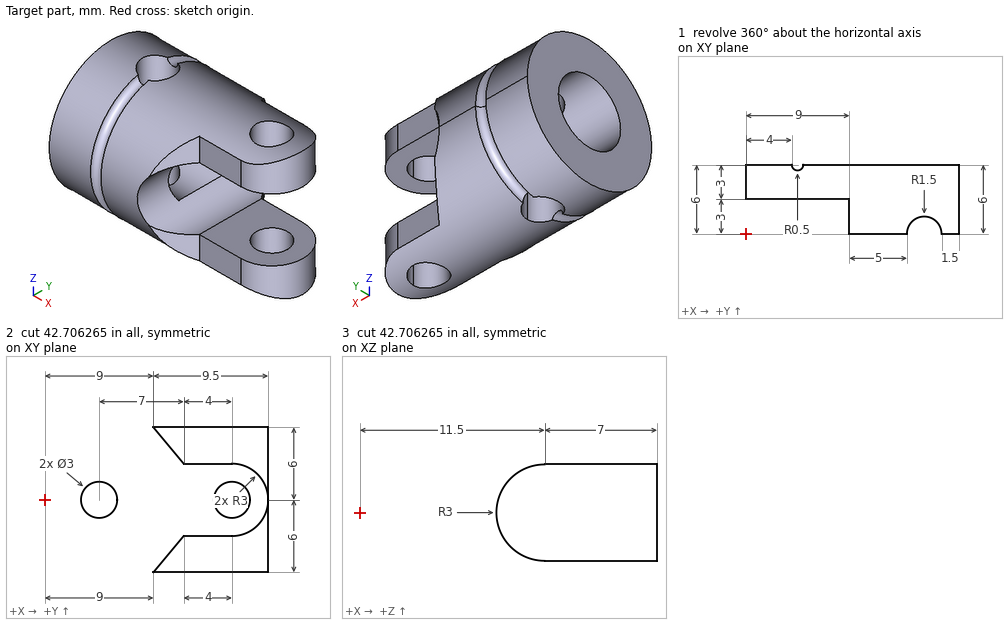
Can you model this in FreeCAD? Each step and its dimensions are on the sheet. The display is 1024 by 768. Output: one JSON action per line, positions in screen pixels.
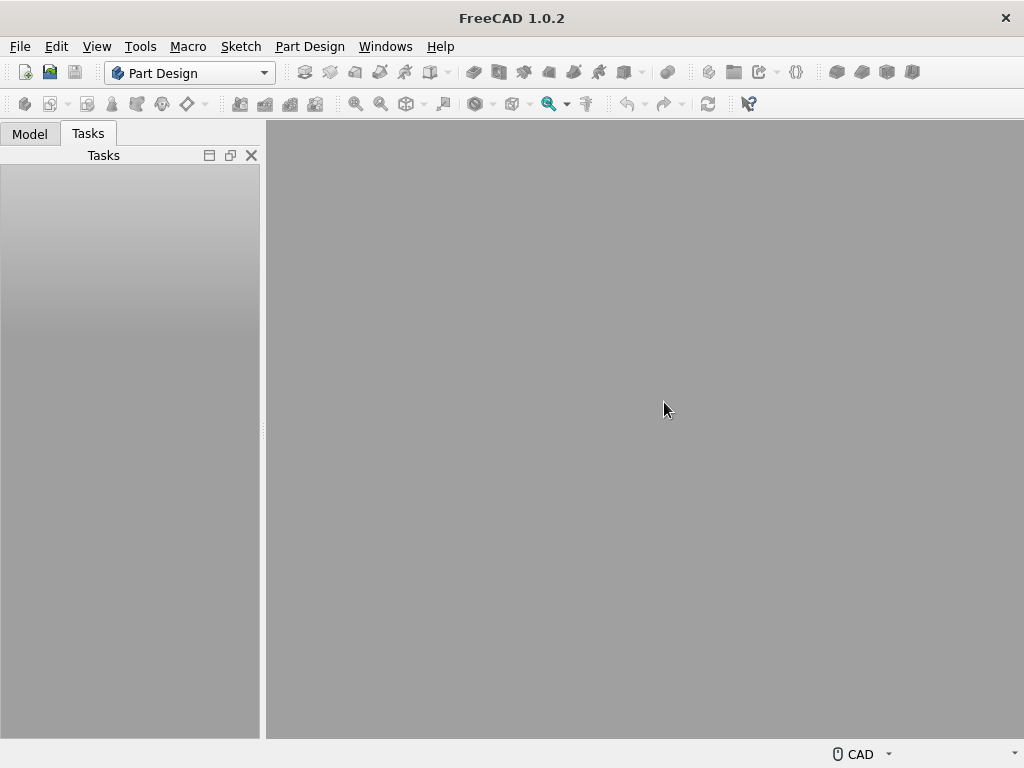
{"action": "left_click", "coordinate": [25, 72]}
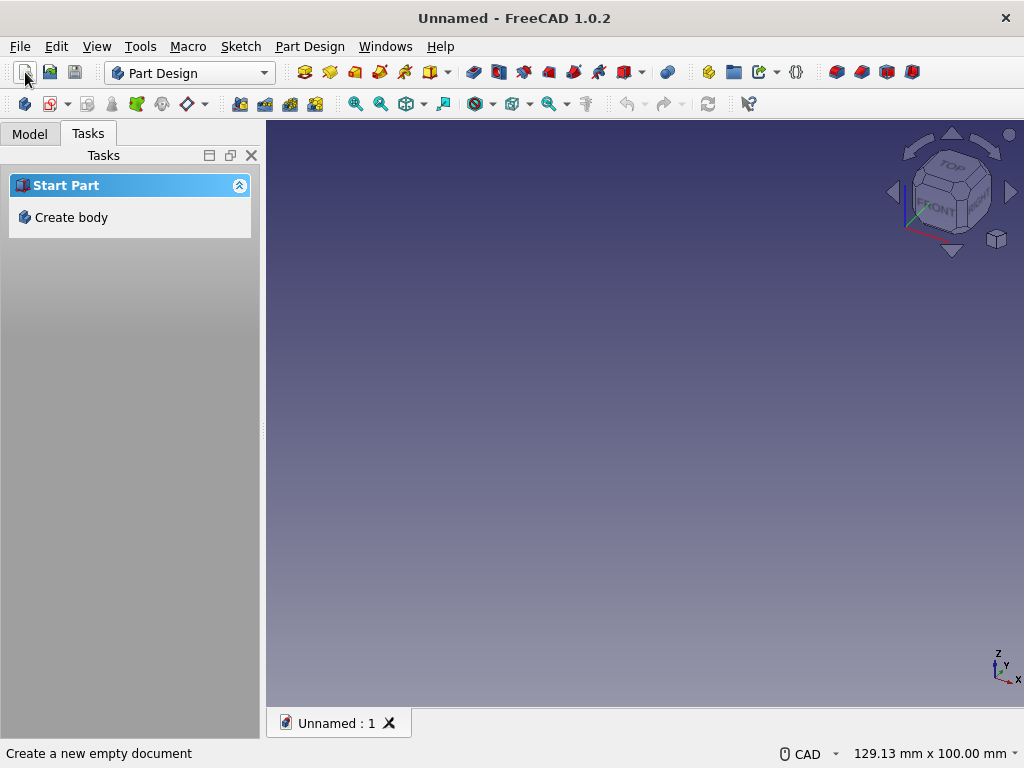
{"action": "left_click", "coordinate": [50, 104]}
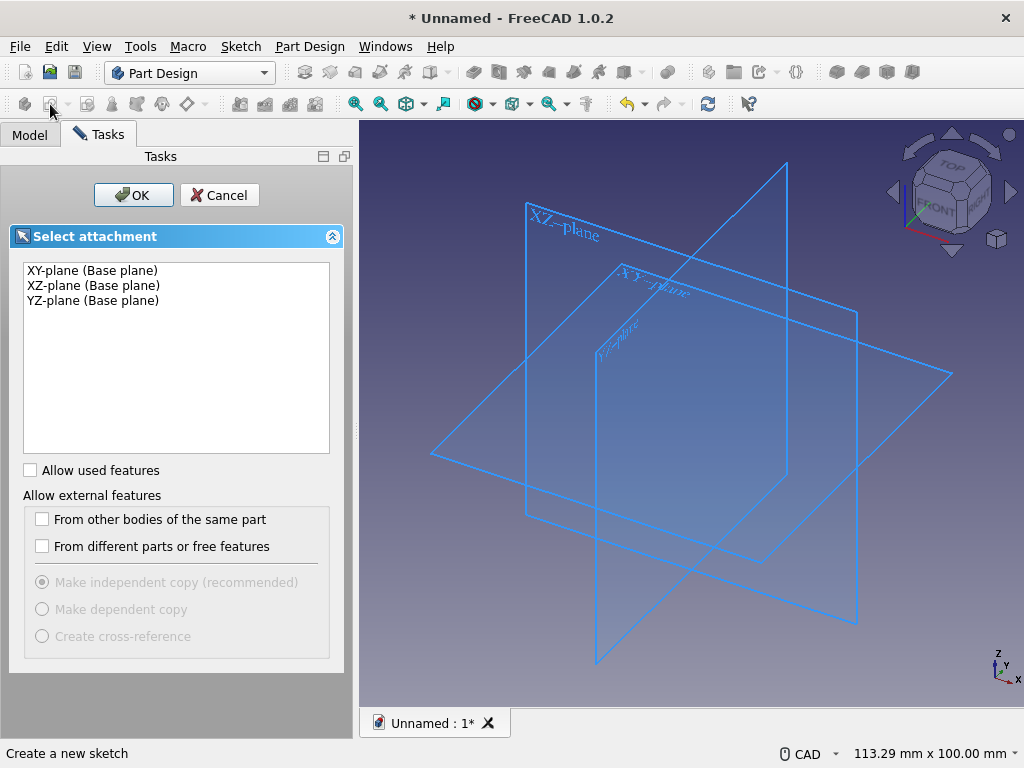
{"action": "left_click", "coordinate": [84, 270]}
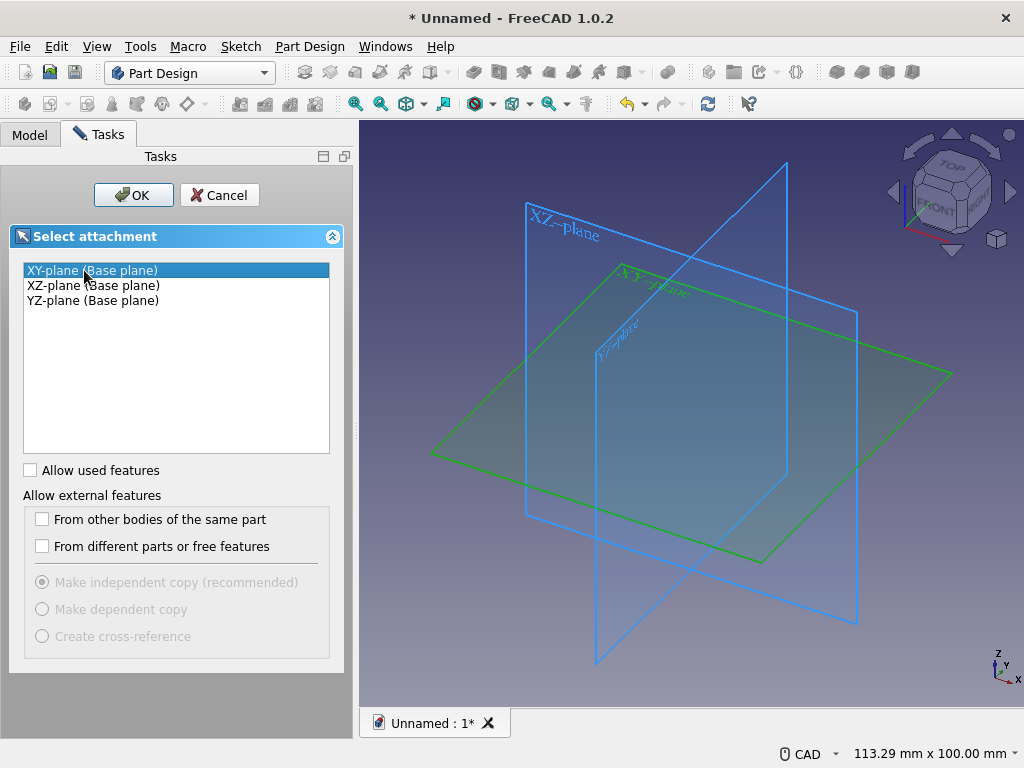
{"action": "left_click", "coordinate": [134, 195]}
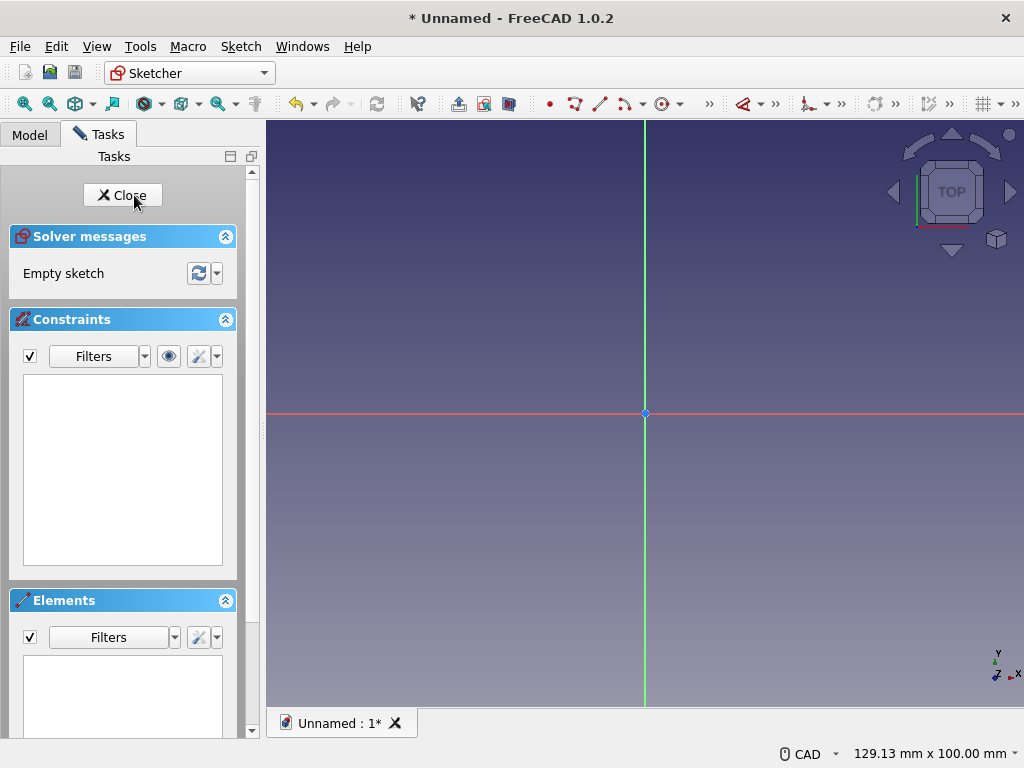
{"action": "scroll", "coordinate": [739, 390], "scroll_direction": "up", "scroll_amount": 7}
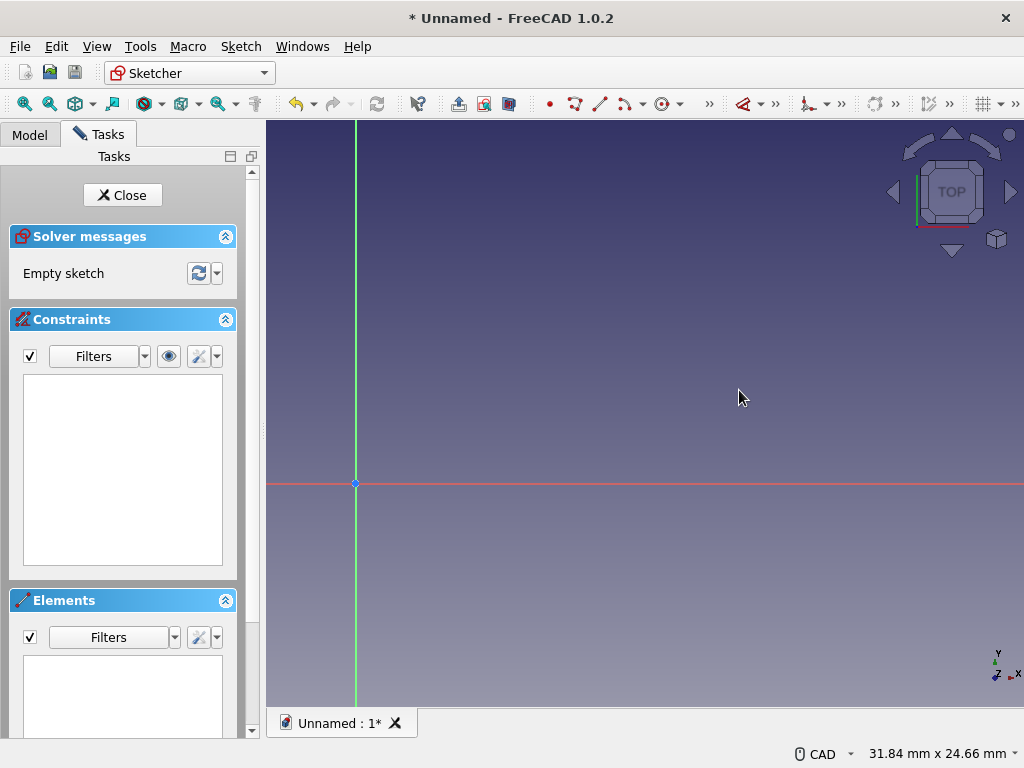
{"action": "left_click", "coordinate": [575, 104]}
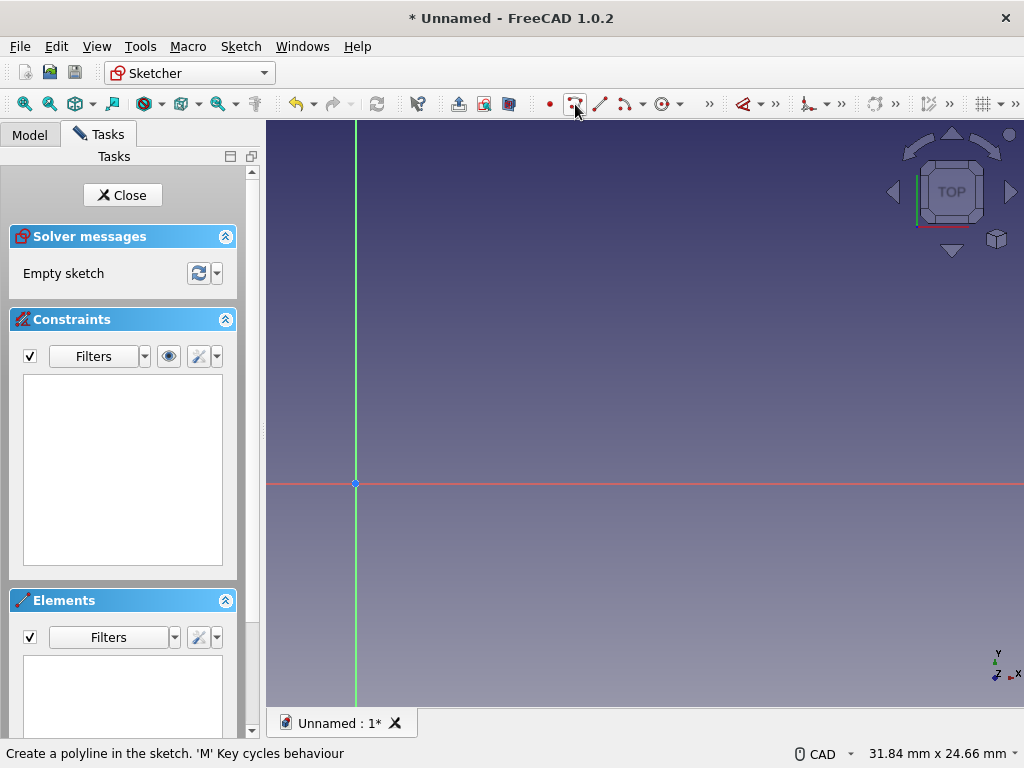
{"action": "left_click", "coordinate": [451, 341]}
{"action": "left_click", "coordinate": [356, 341]}
{"action": "left_click", "coordinate": [365, 412]}
{"action": "left_click", "coordinate": [570, 412]}
{"action": "left_click", "coordinate": [570, 484]}
{"action": "left_click", "coordinate": [689, 475]}
{"action": "right_click", "coordinate": [689, 475]}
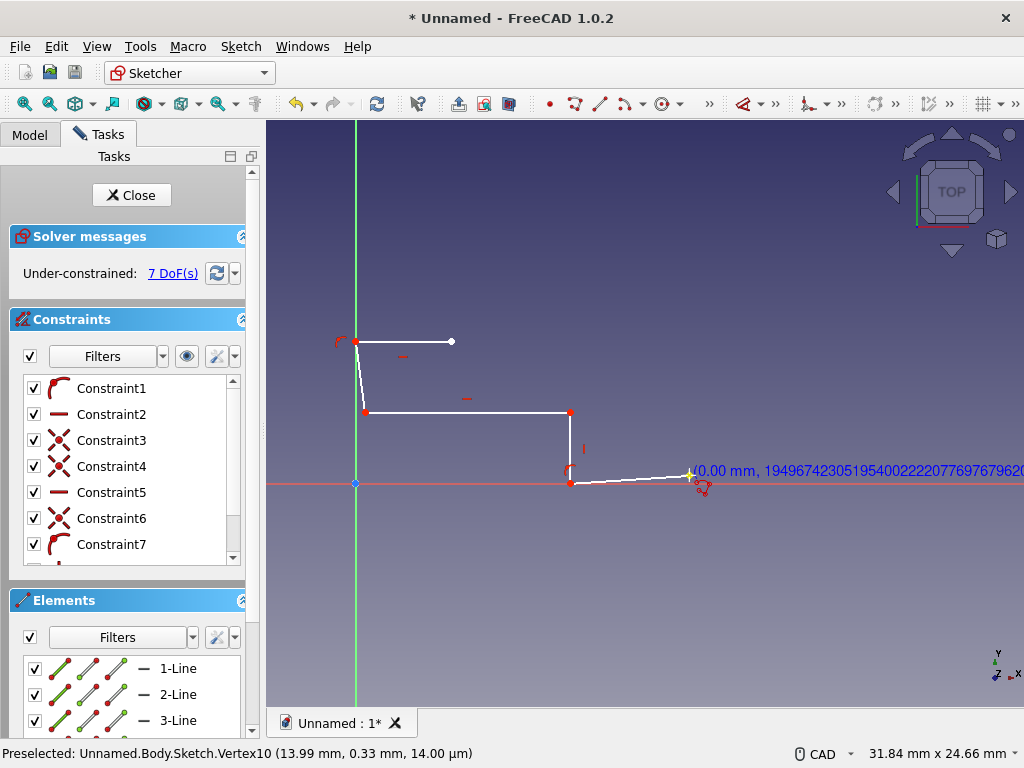
{"action": "left_click", "coordinate": [761, 484]}
{"action": "left_click", "coordinate": [796, 475]}
{"action": "left_click", "coordinate": [796, 341]}
{"action": "left_click", "coordinate": [475, 341]}
{"action": "right_click", "coordinate": [475, 341]}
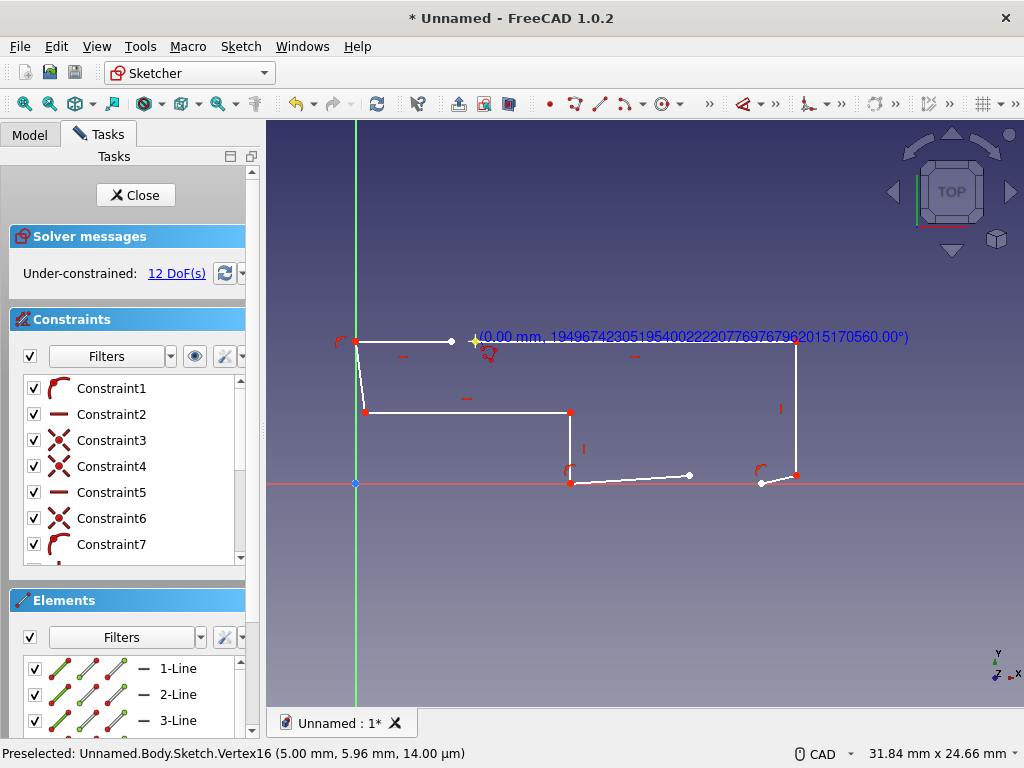
{"action": "key", "text": "g 3 a"}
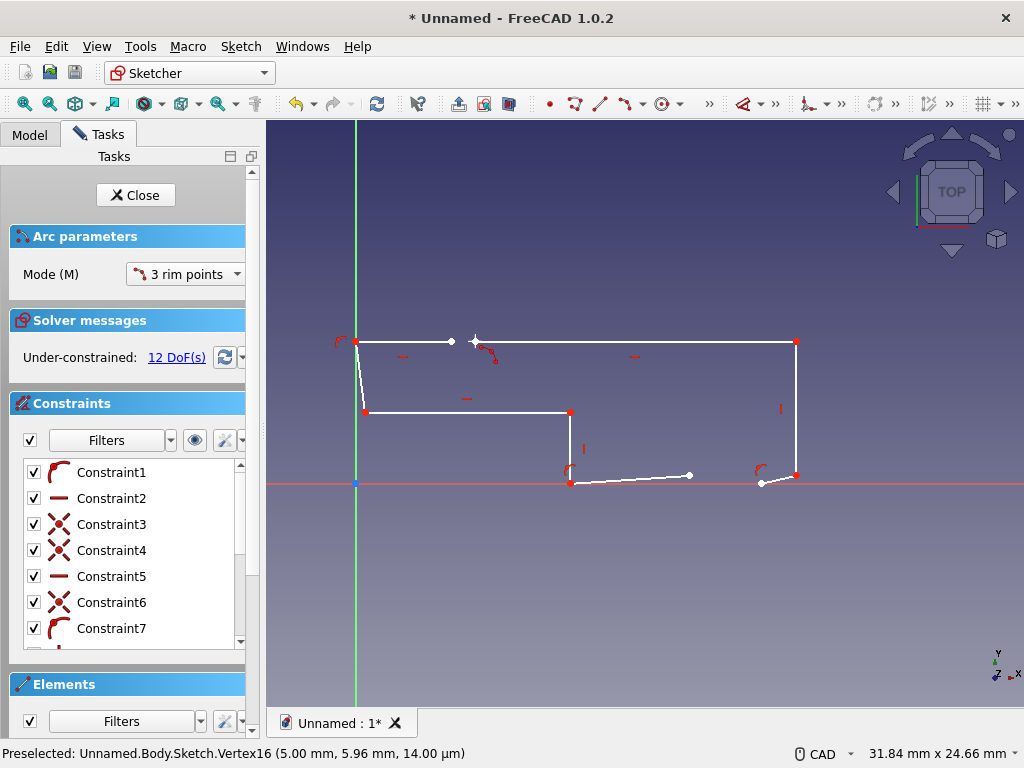
{"action": "left_click", "coordinate": [689, 476]}
{"action": "left_click", "coordinate": [761, 484]}
{"action": "left_click", "coordinate": [725, 448]}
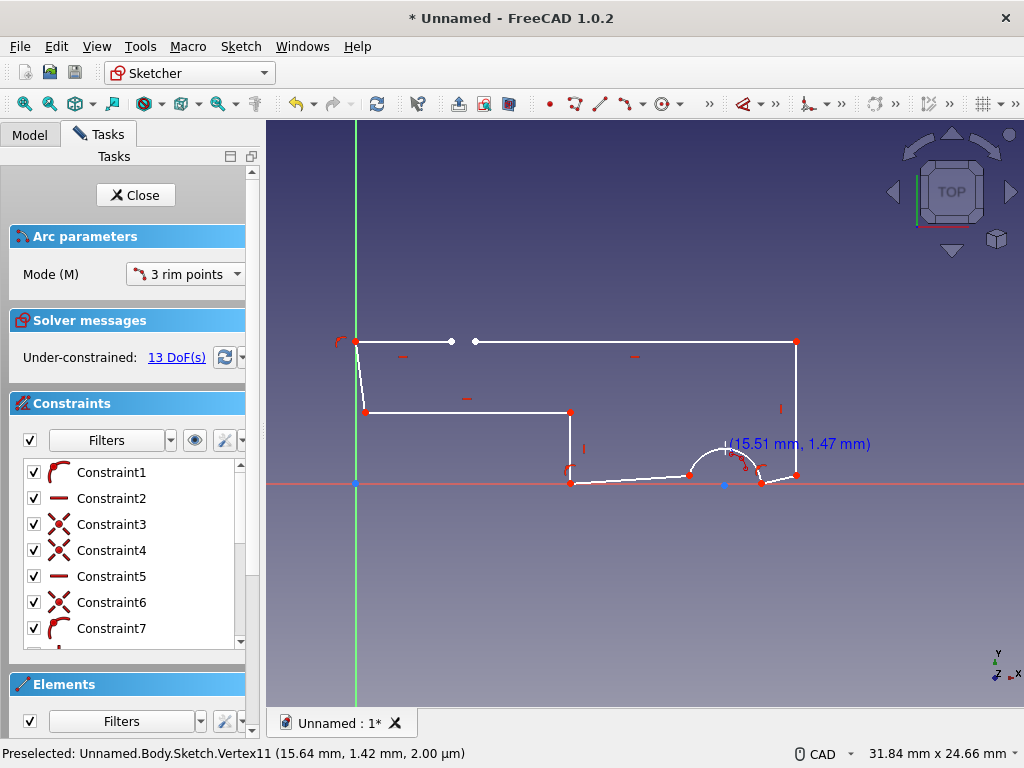
{"action": "left_click", "coordinate": [475, 342]}
{"action": "left_click", "coordinate": [451, 342]}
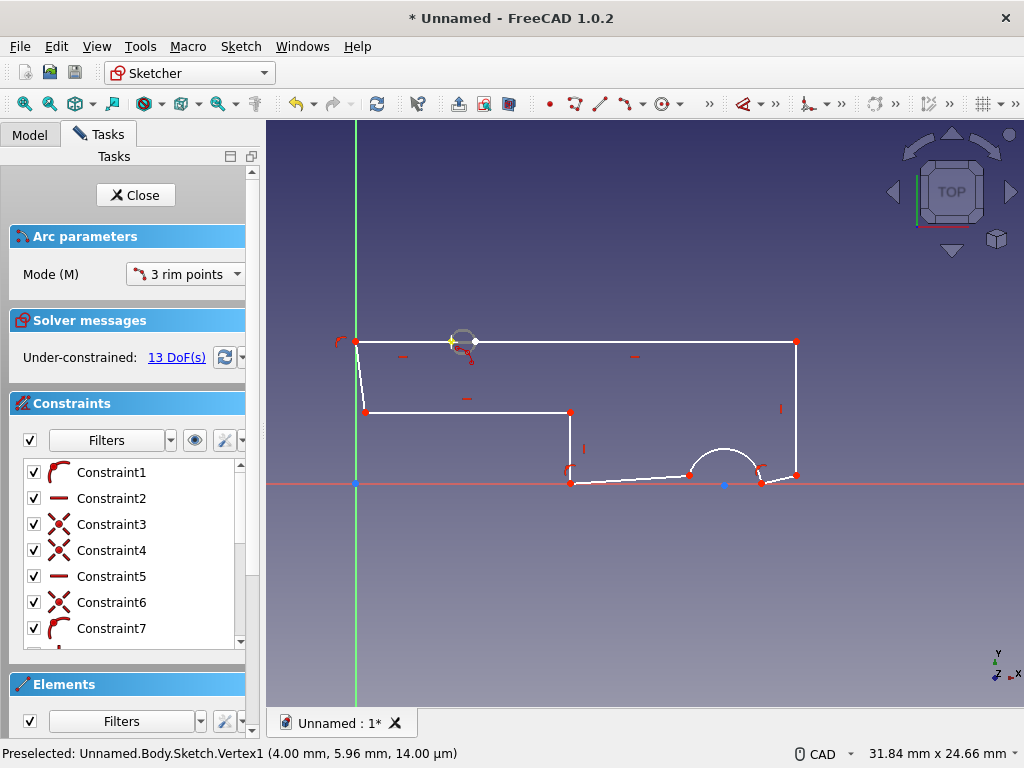
{"action": "scroll", "coordinate": [463, 353], "scroll_direction": "up", "scroll_amount": 2}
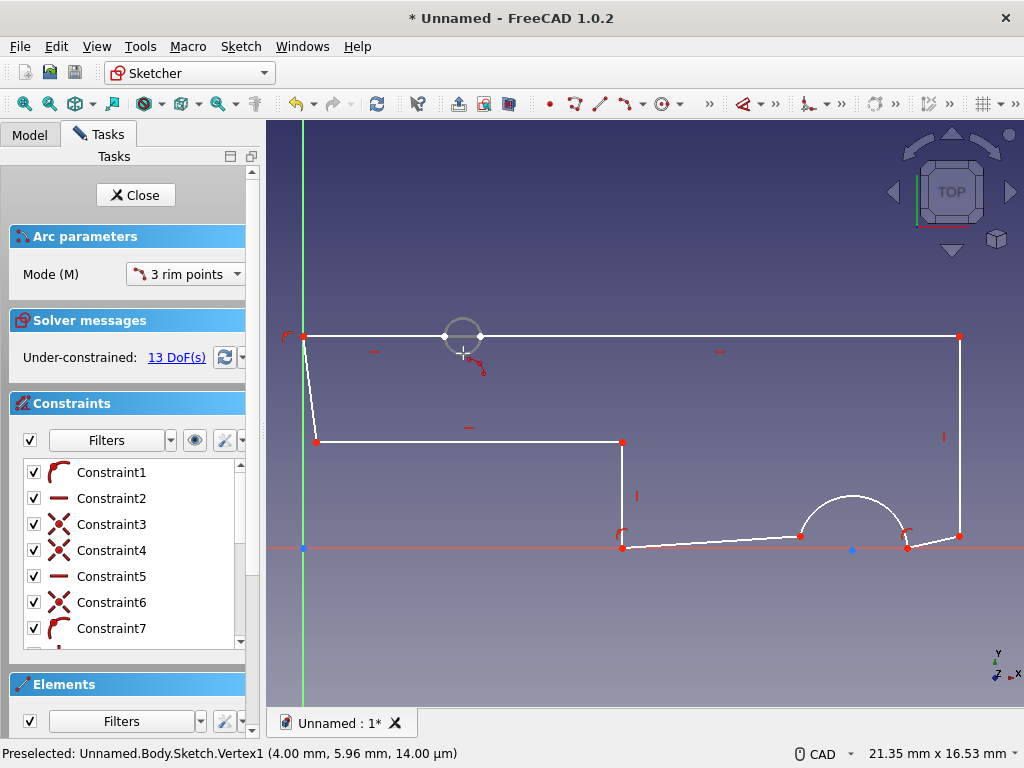
{"action": "left_click", "coordinate": [463, 353]}
{"action": "key", "text": "Escape"}